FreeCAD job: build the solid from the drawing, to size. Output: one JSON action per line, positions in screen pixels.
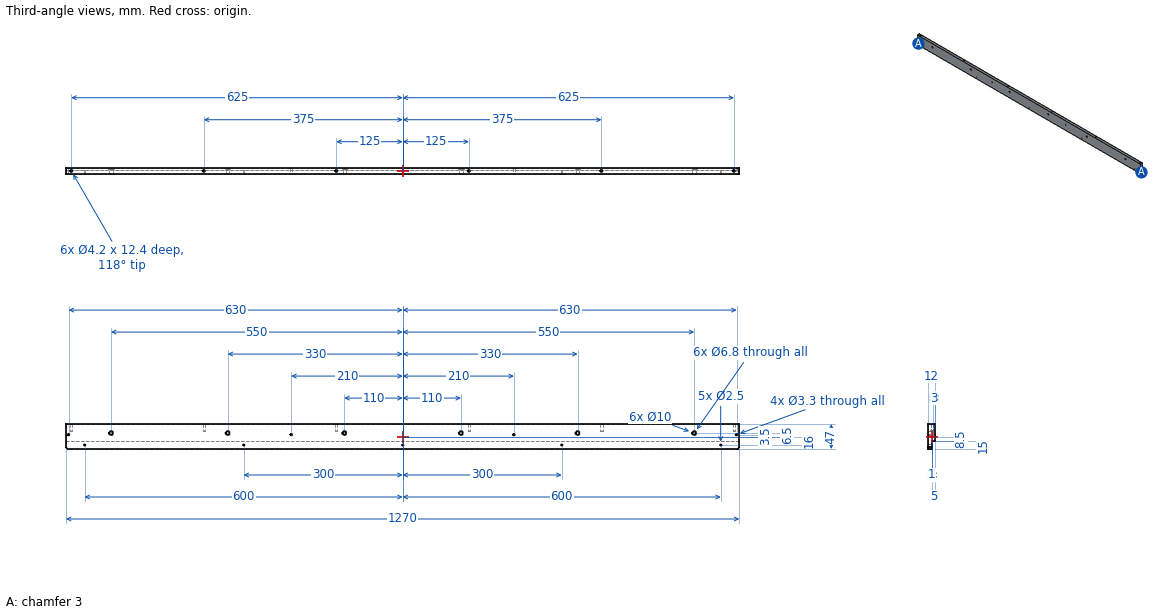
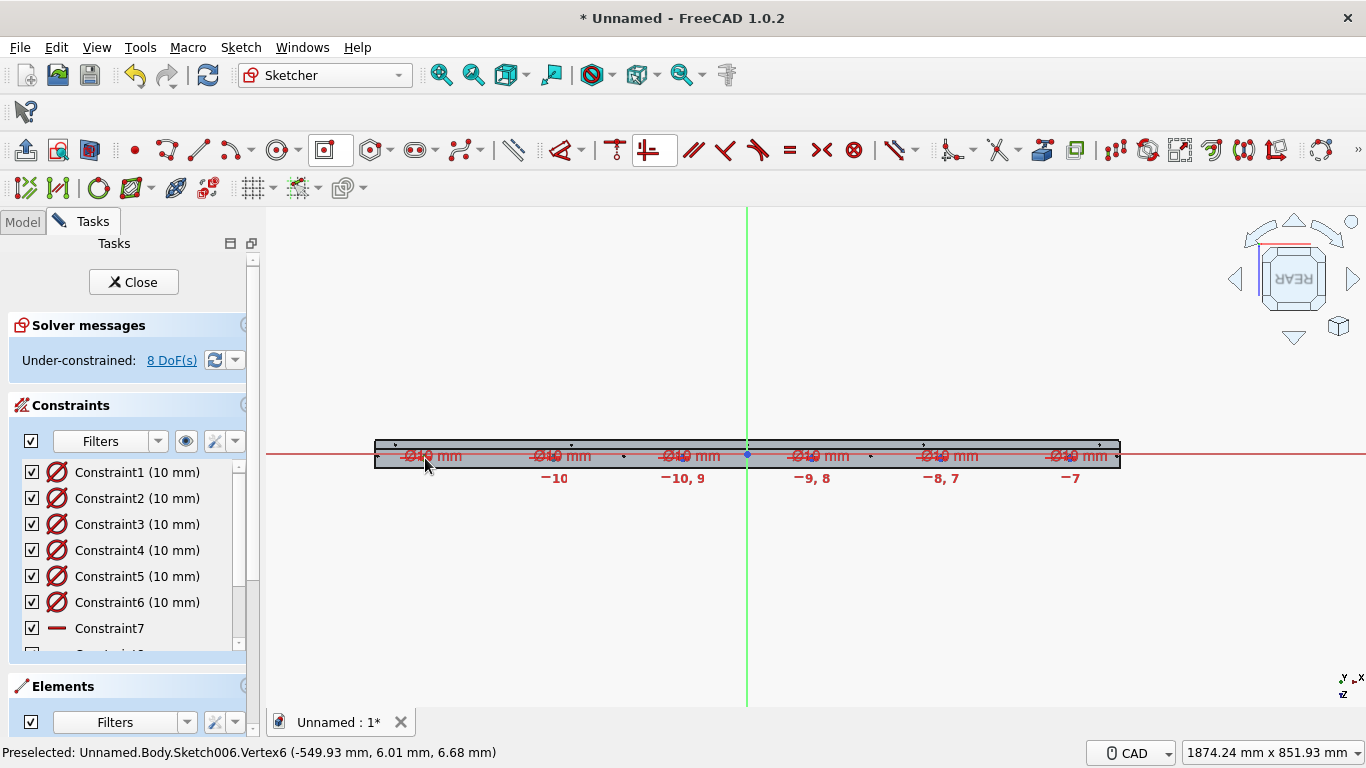
{"action": "key", "text": "h"}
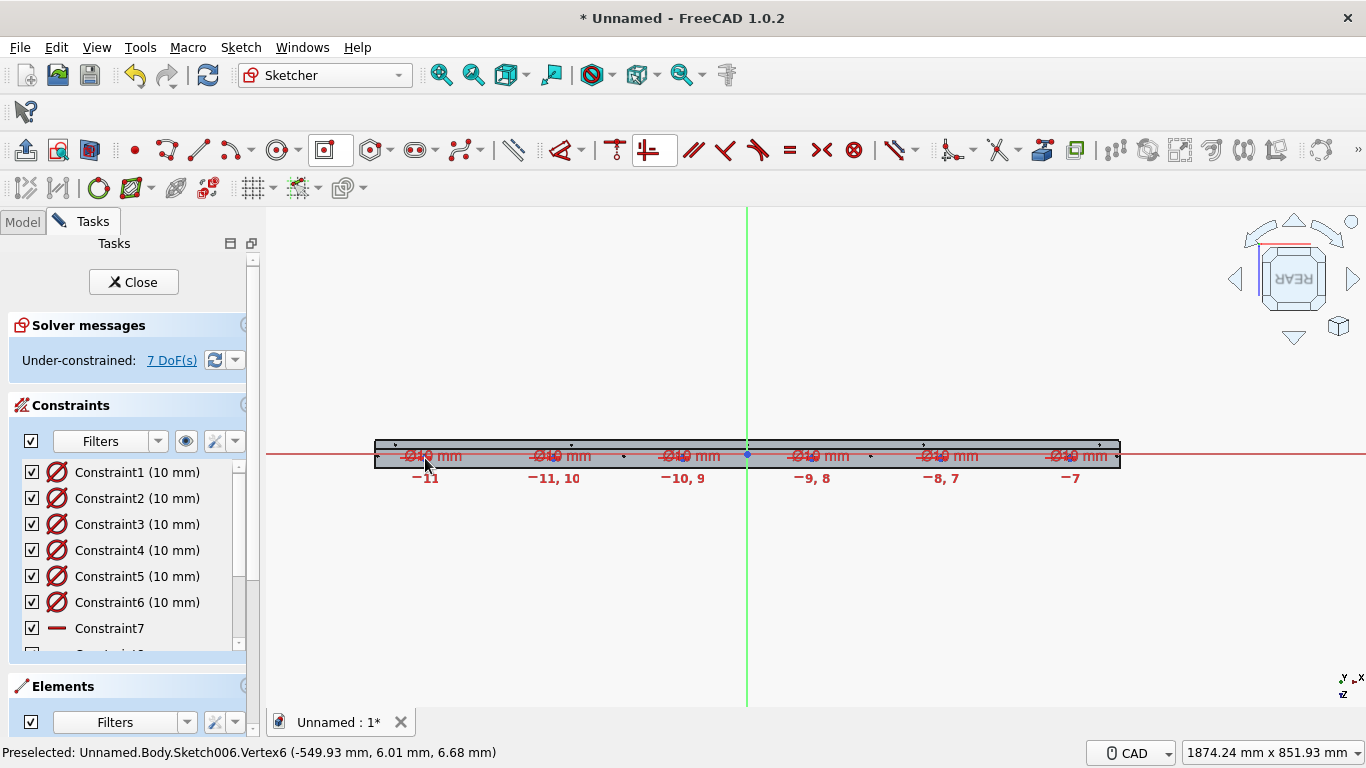
{"action": "left_click", "coordinate": [560, 150]}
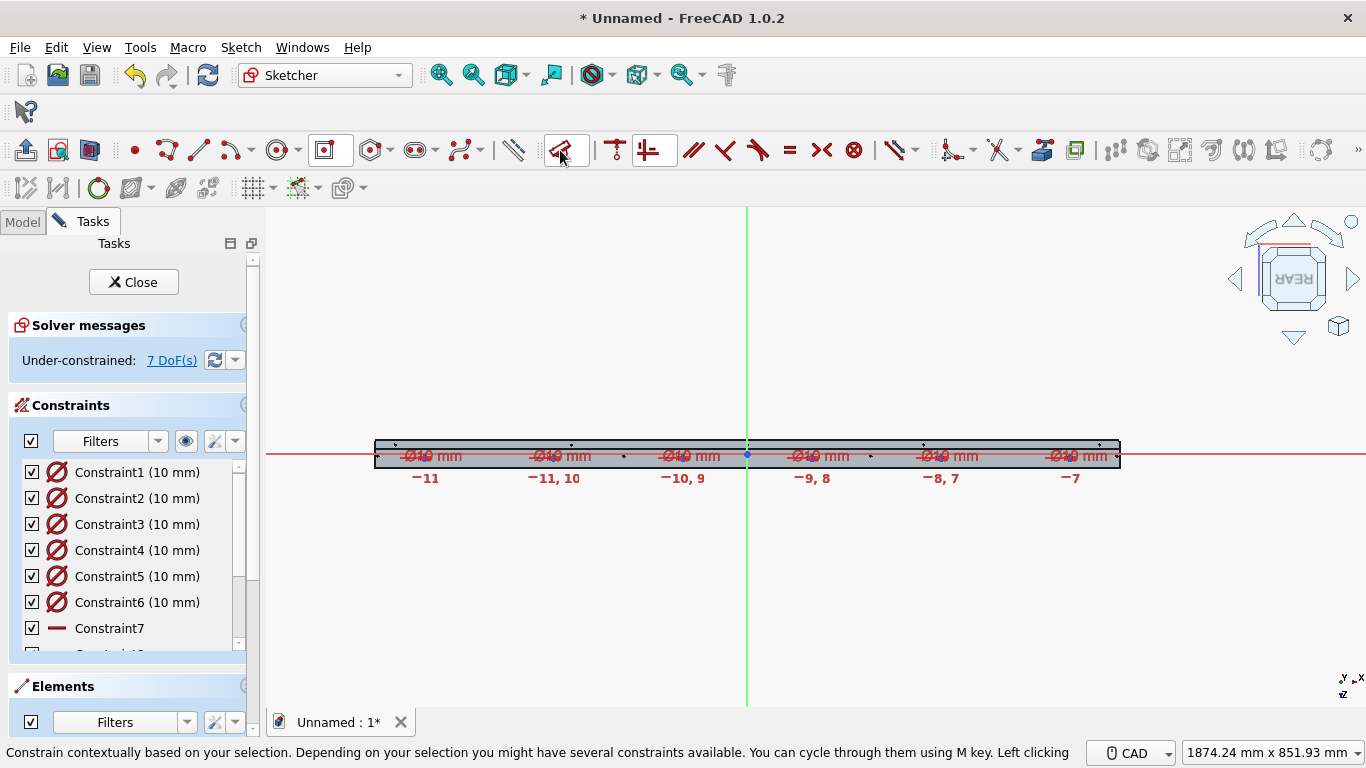
{"action": "left_click", "coordinate": [1070, 458]}
{"action": "left_click", "coordinate": [909, 420]}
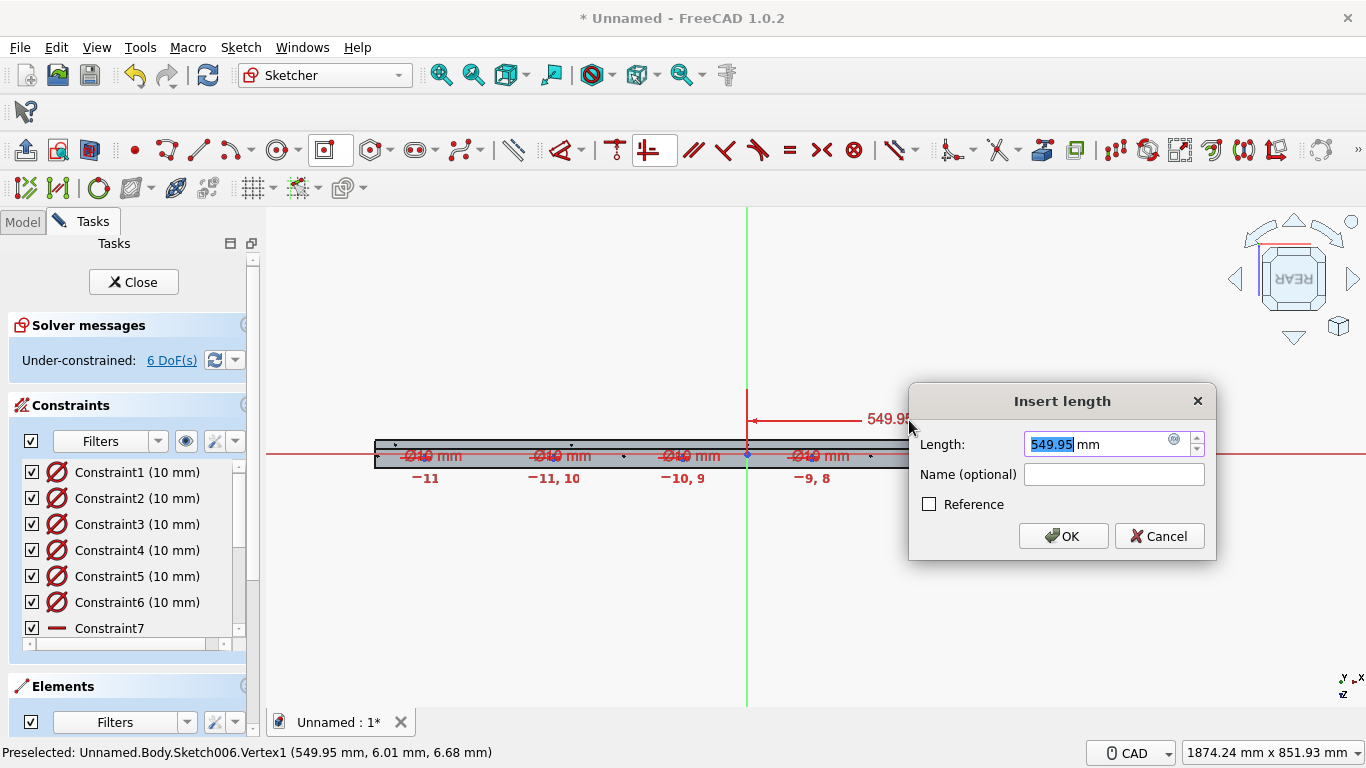
{"action": "type", "text": "550"}
{"action": "key", "text": "Return"}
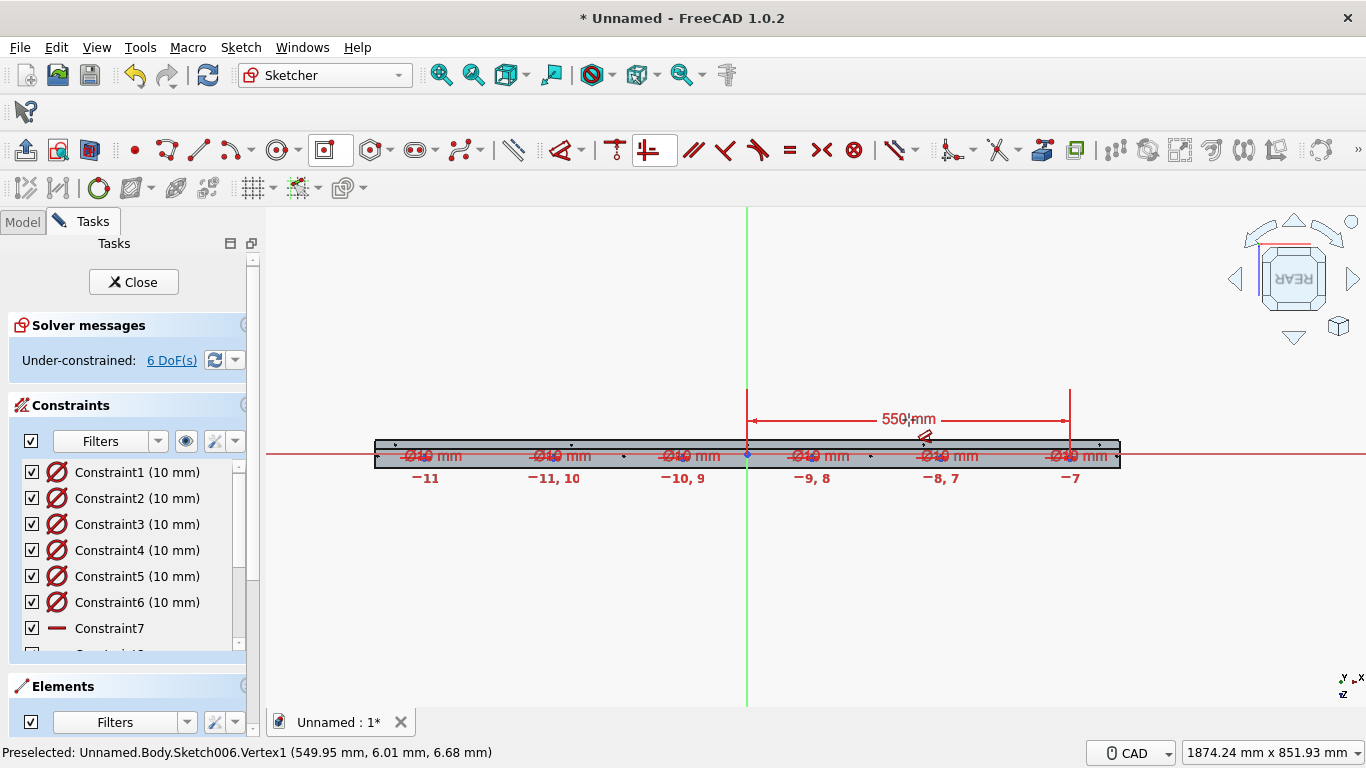
{"action": "scroll", "coordinate": [1070, 458], "scroll_direction": "up", "scroll_amount": 12}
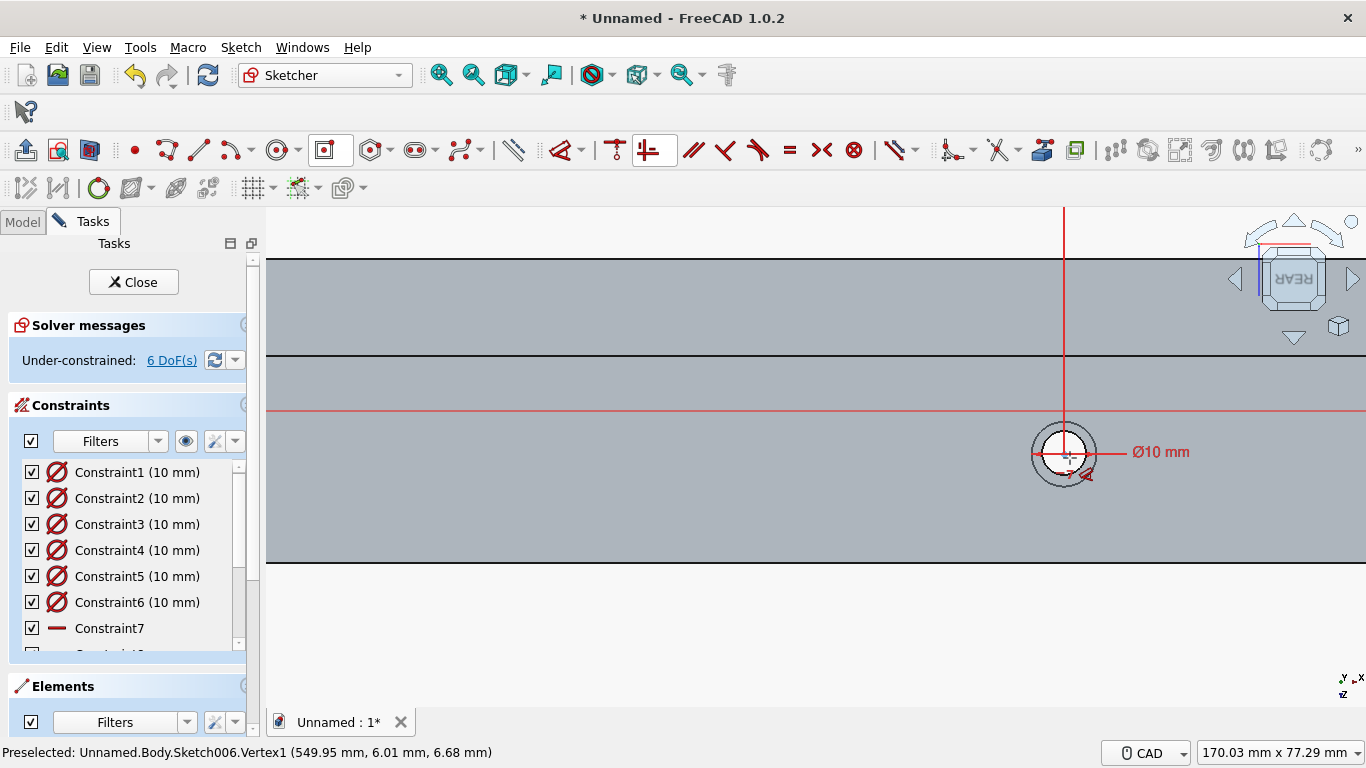
{"action": "left_click", "coordinate": [1064, 454]}
{"action": "left_click", "coordinate": [1122, 433]}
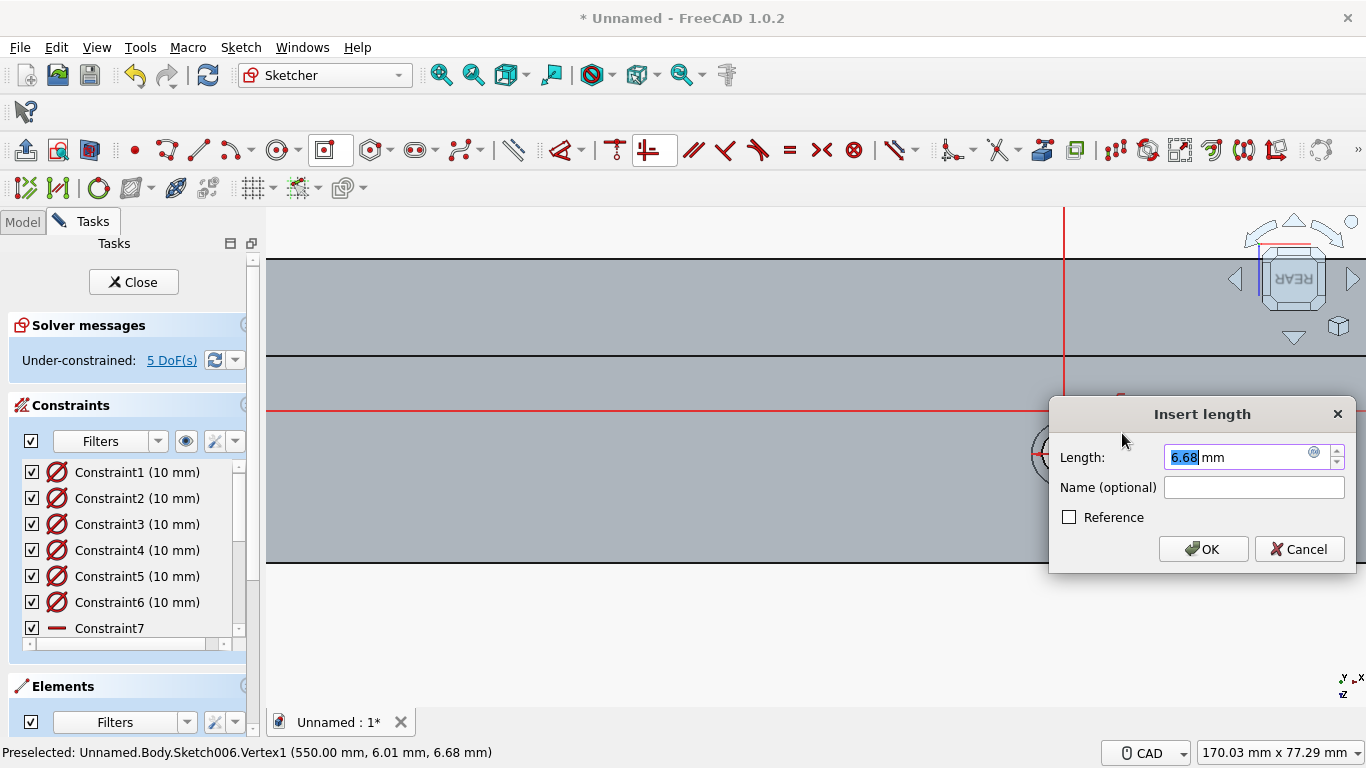
{"action": "type", "text": "6.5"}
{"action": "key", "text": "Return"}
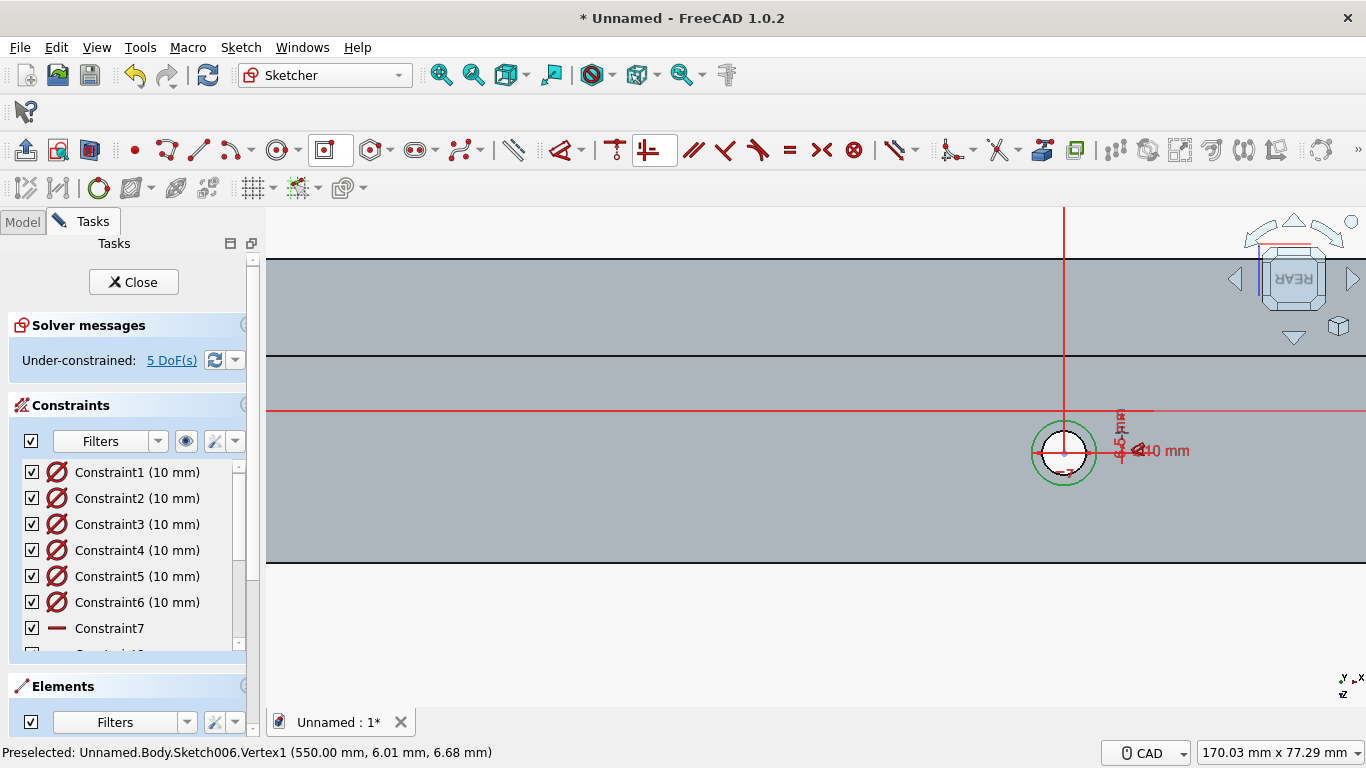
{"action": "scroll", "coordinate": [1071, 458], "scroll_direction": "down", "scroll_amount": 12}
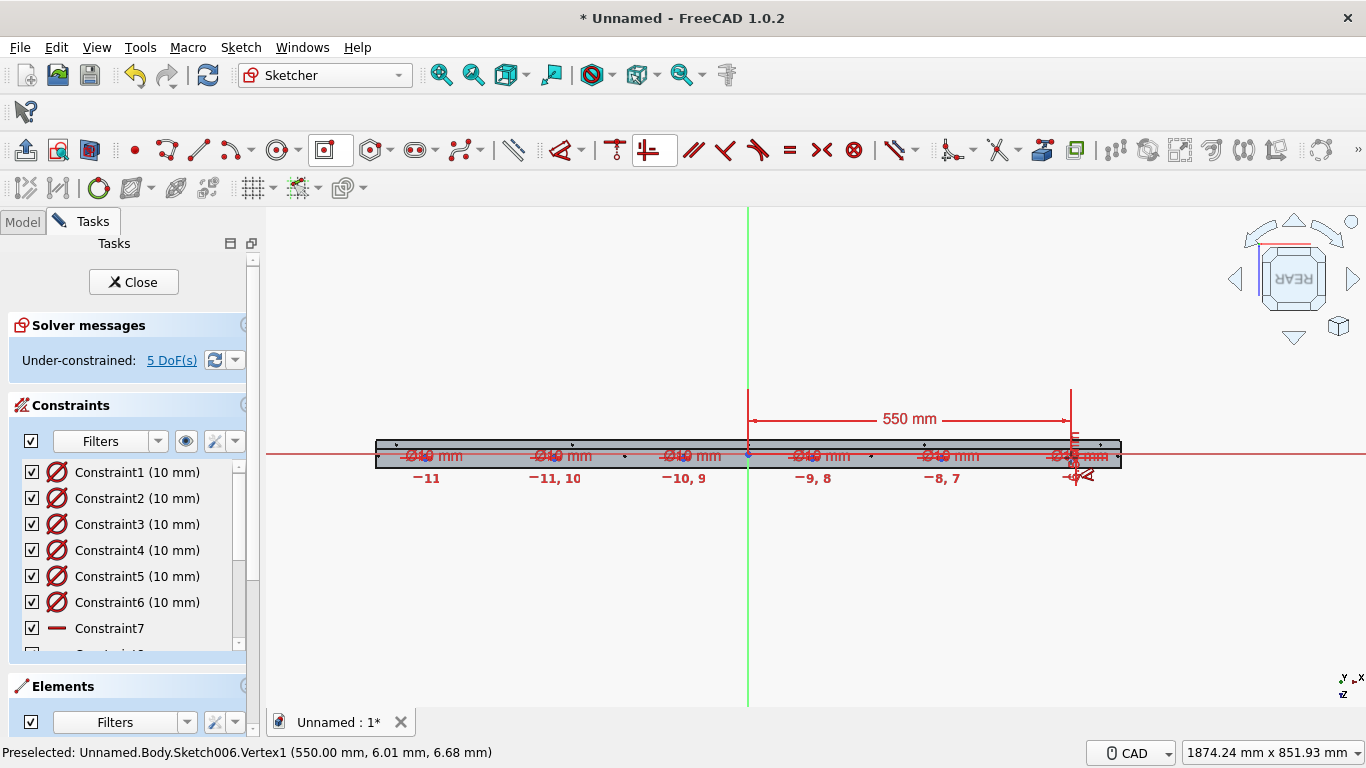
{"action": "left_click", "coordinate": [942, 458]}
{"action": "left_click", "coordinate": [801, 420]}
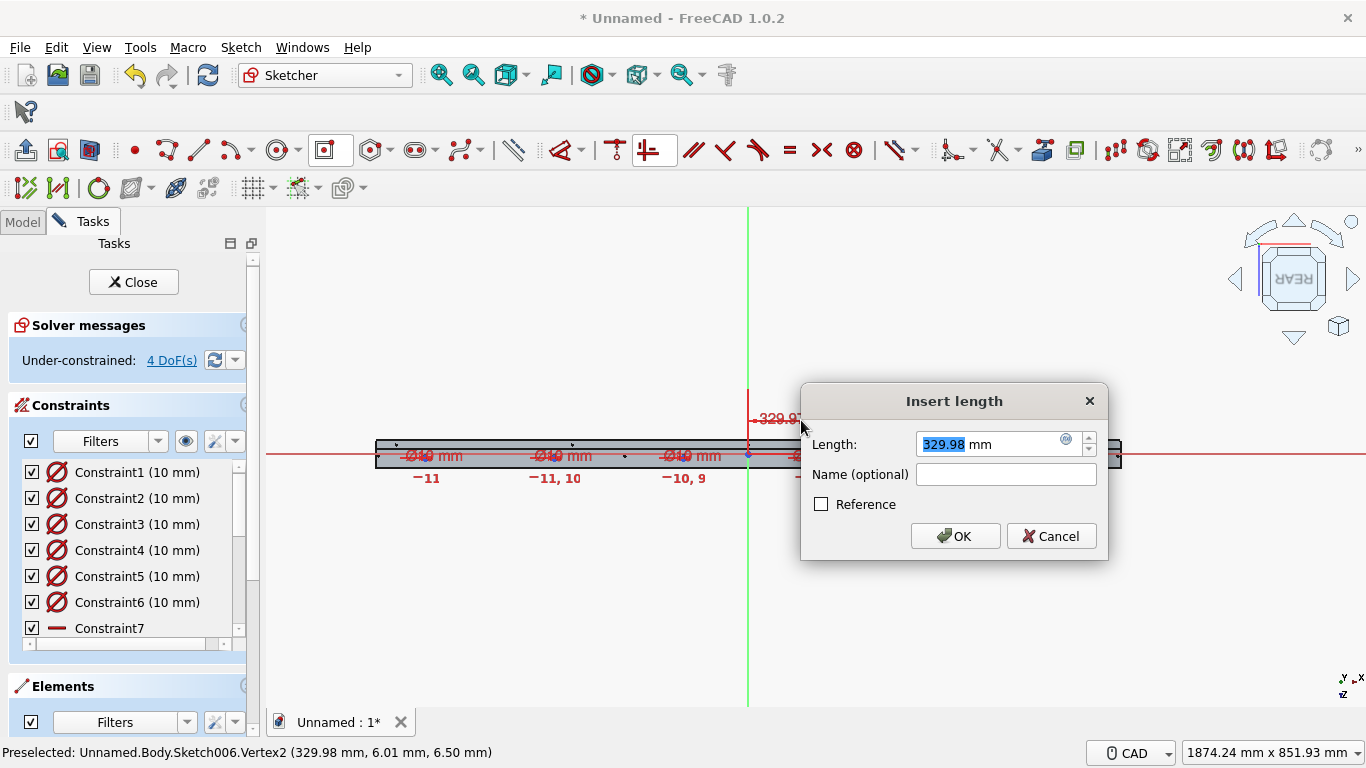
{"action": "type", "text": "330"}
{"action": "key", "text": "Return"}